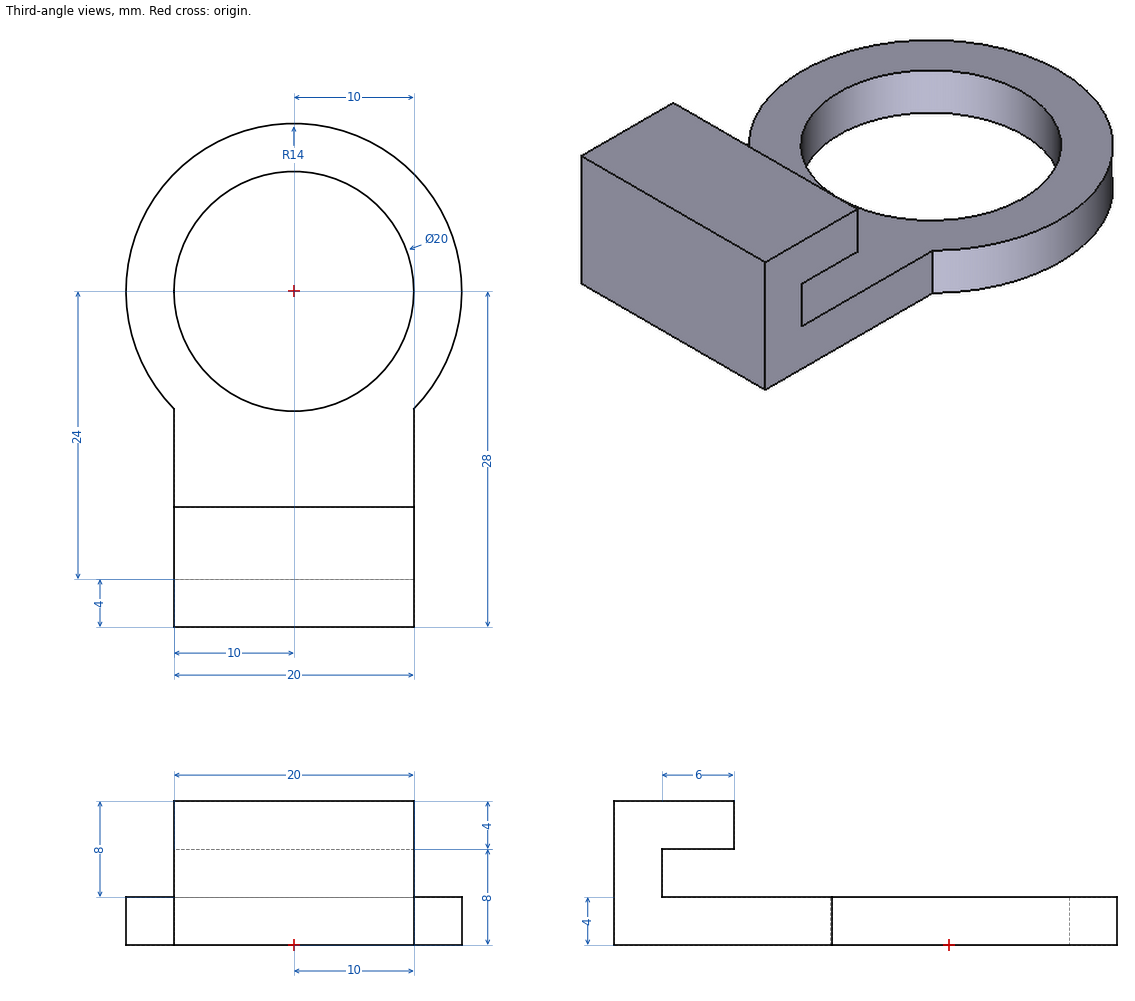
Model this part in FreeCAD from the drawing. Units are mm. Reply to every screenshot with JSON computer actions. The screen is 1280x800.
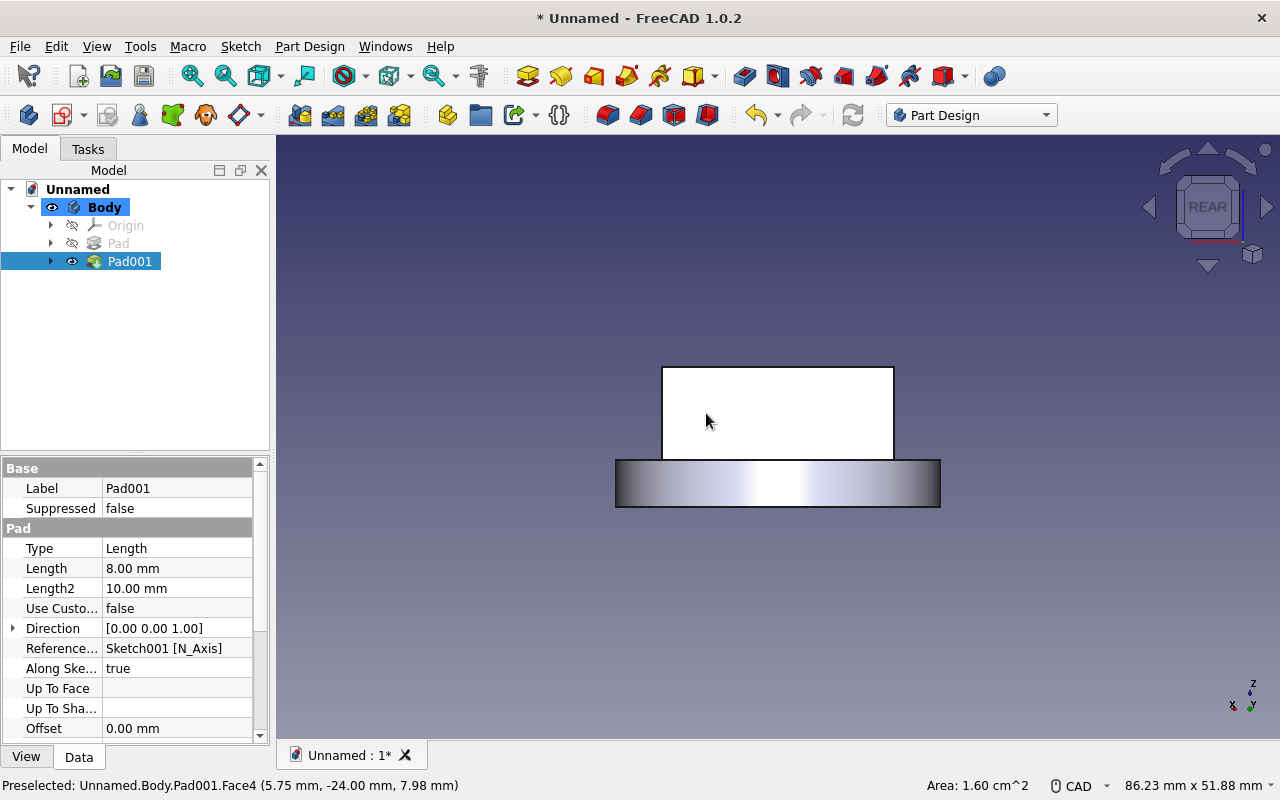
{"action": "left_click", "coordinate": [62, 116]}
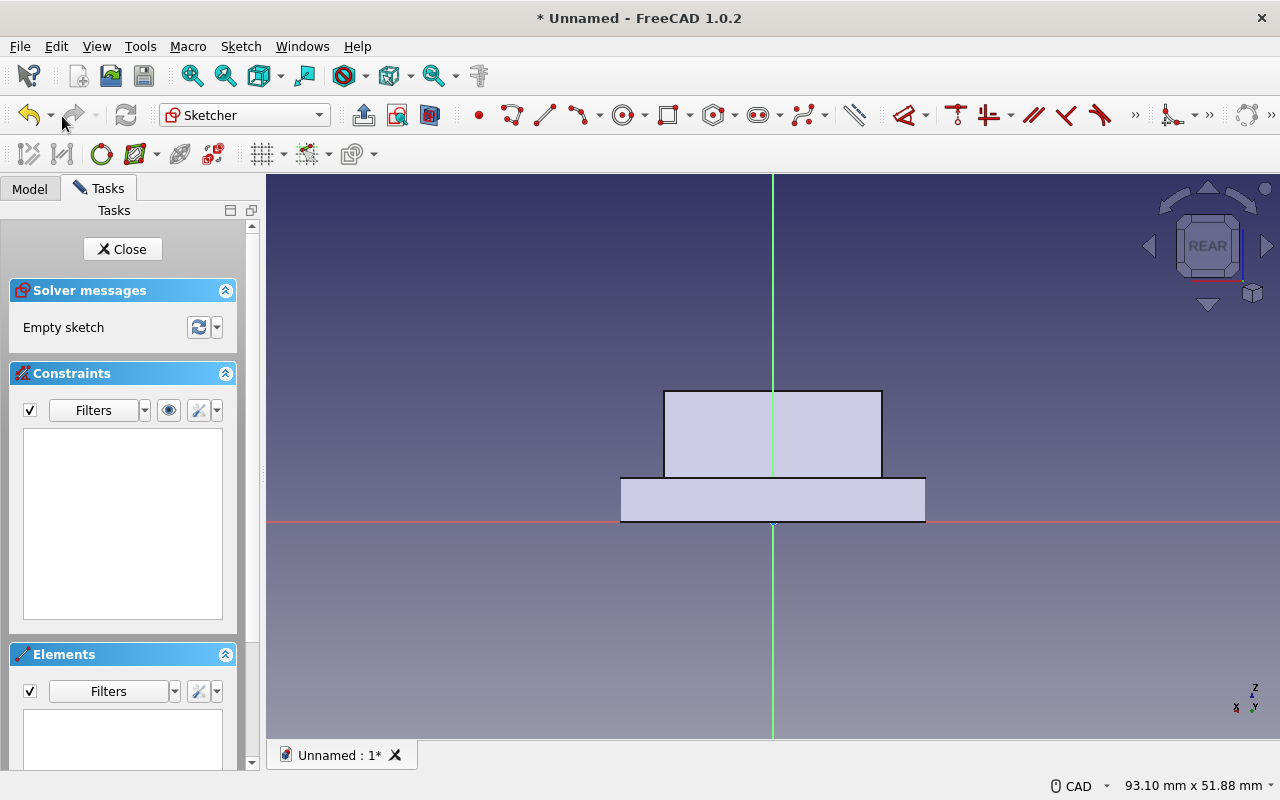
{"action": "left_click", "coordinate": [430, 116]}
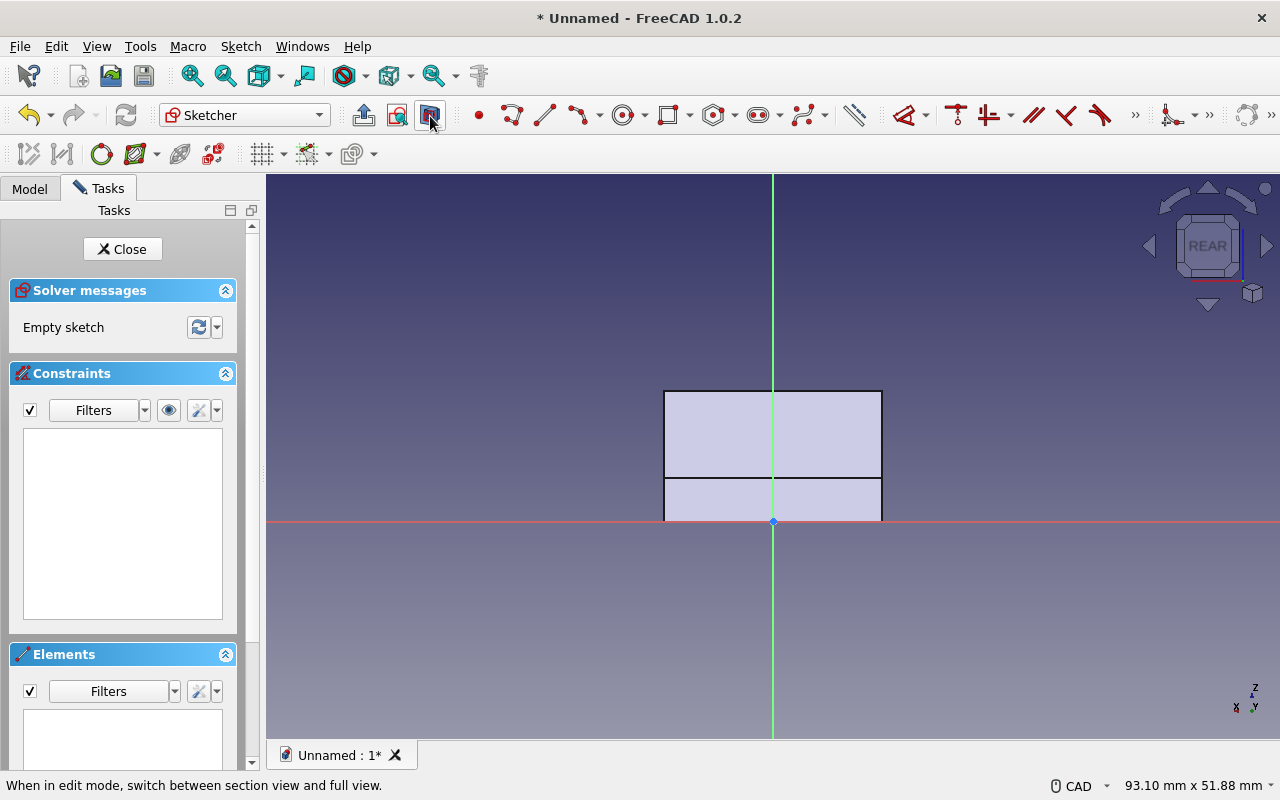
{"action": "scroll", "coordinate": [813, 456], "scroll_direction": "up", "scroll_amount": 5}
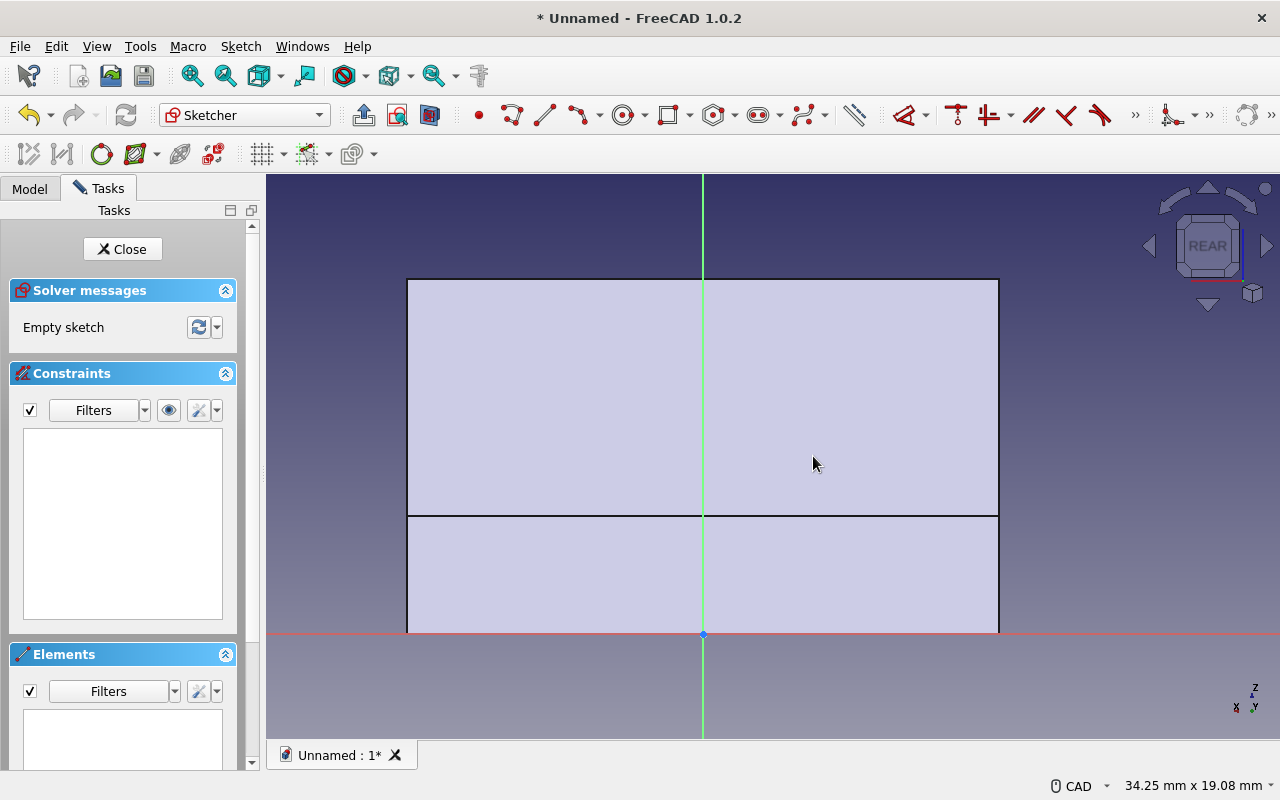
{"action": "left_click", "coordinate": [668, 116]}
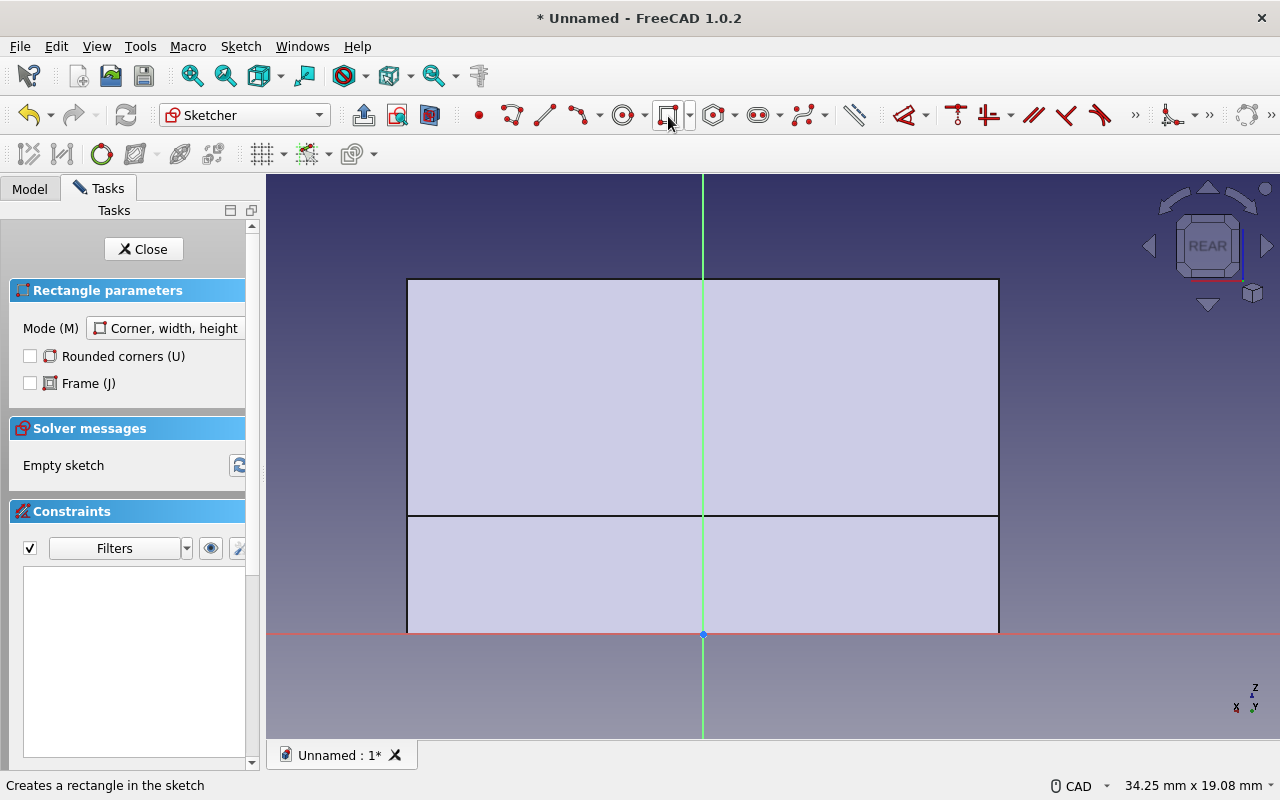
{"action": "left_click", "coordinate": [407, 279]}
{"action": "left_click", "coordinate": [999, 397]}
{"action": "key", "text": "Escape"}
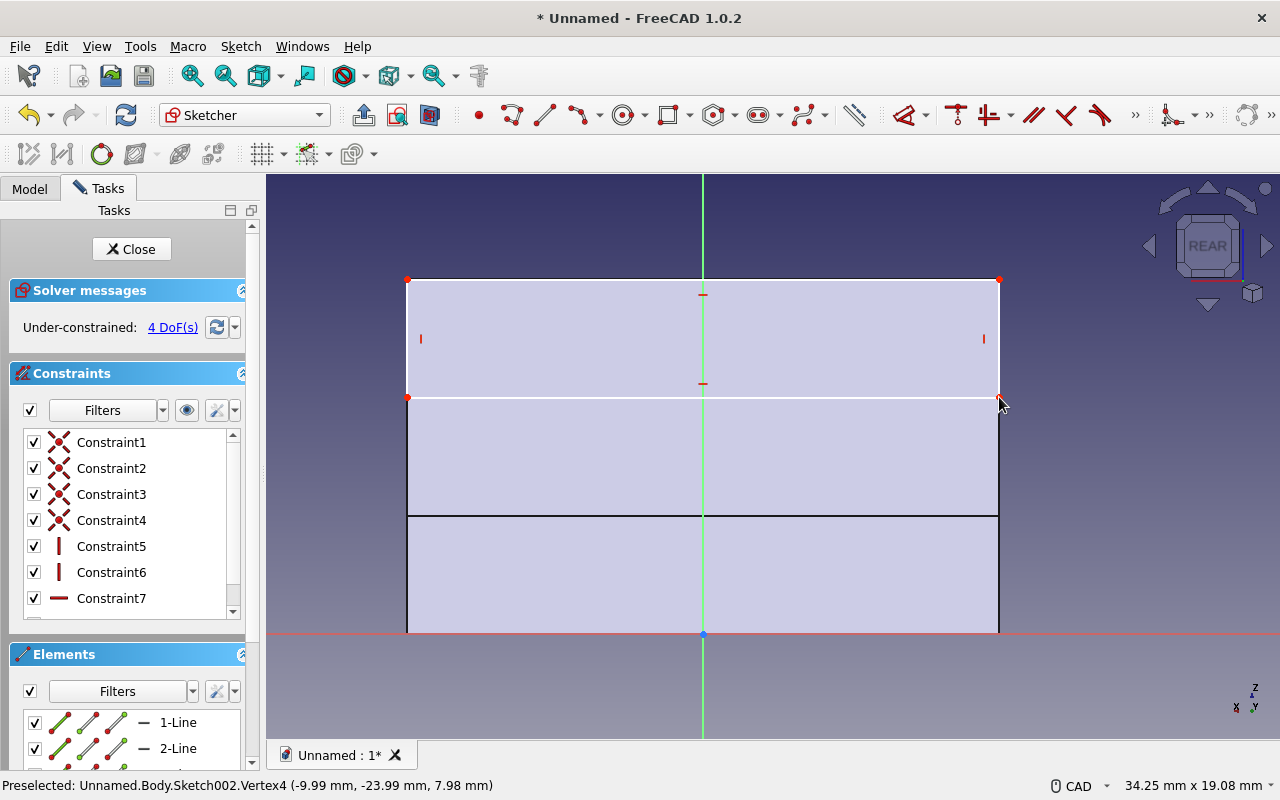
{"action": "key", "text": "d"}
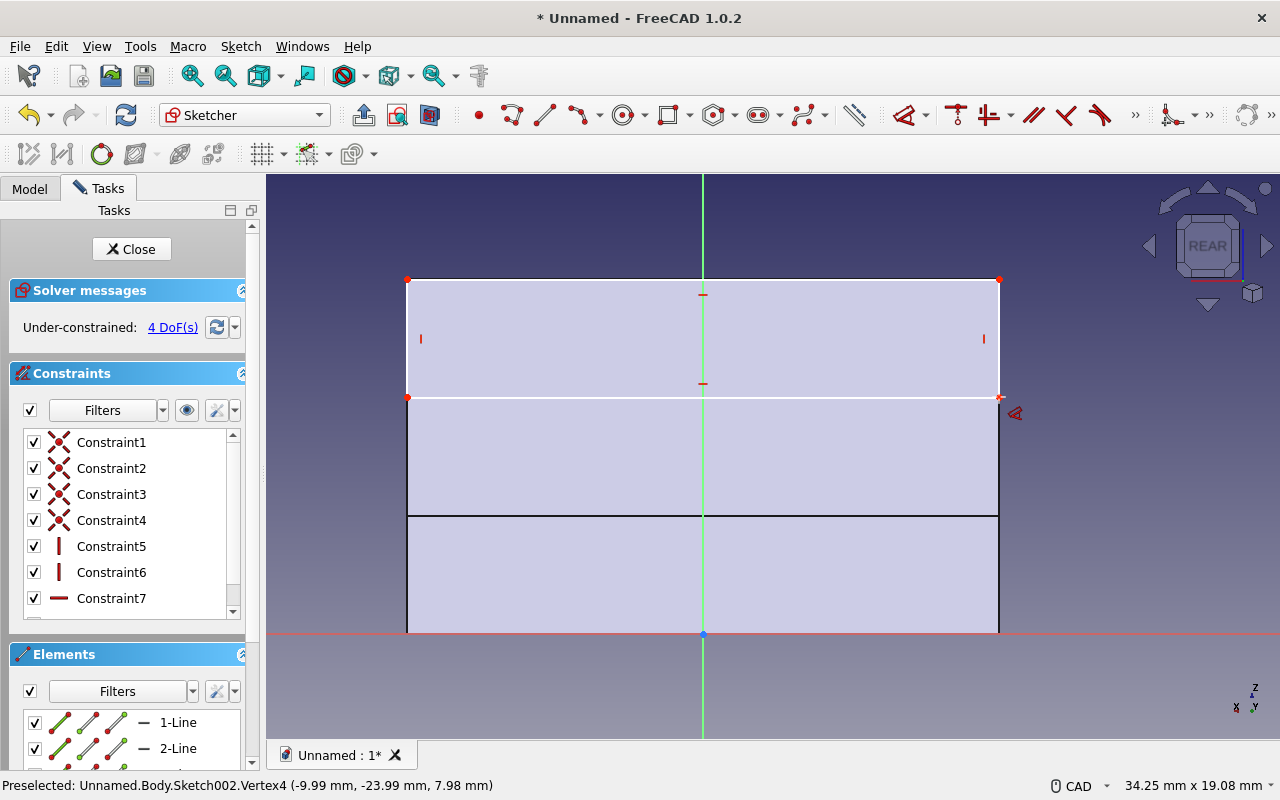
{"action": "left_click", "coordinate": [407, 315]}
{"action": "left_click", "coordinate": [373, 339]}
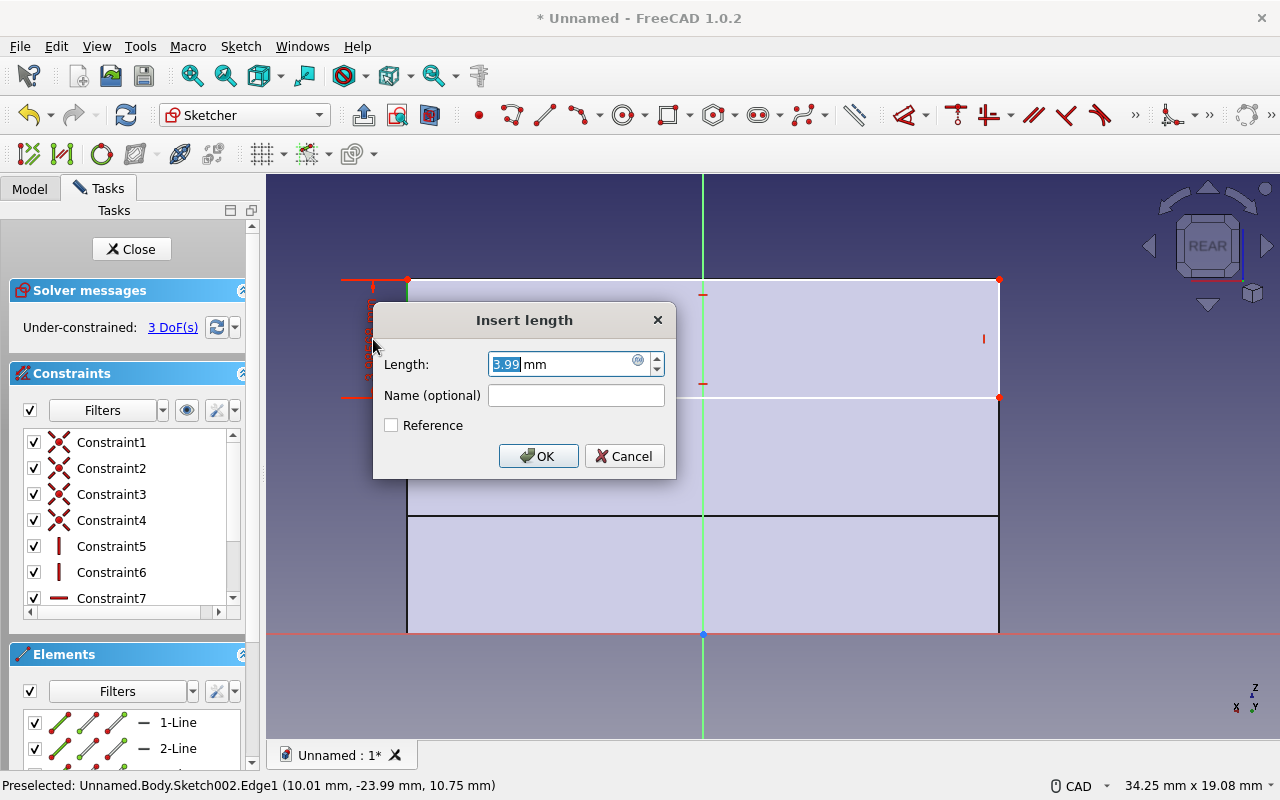
{"action": "type", "text": "4"}
{"action": "key", "text": "Return"}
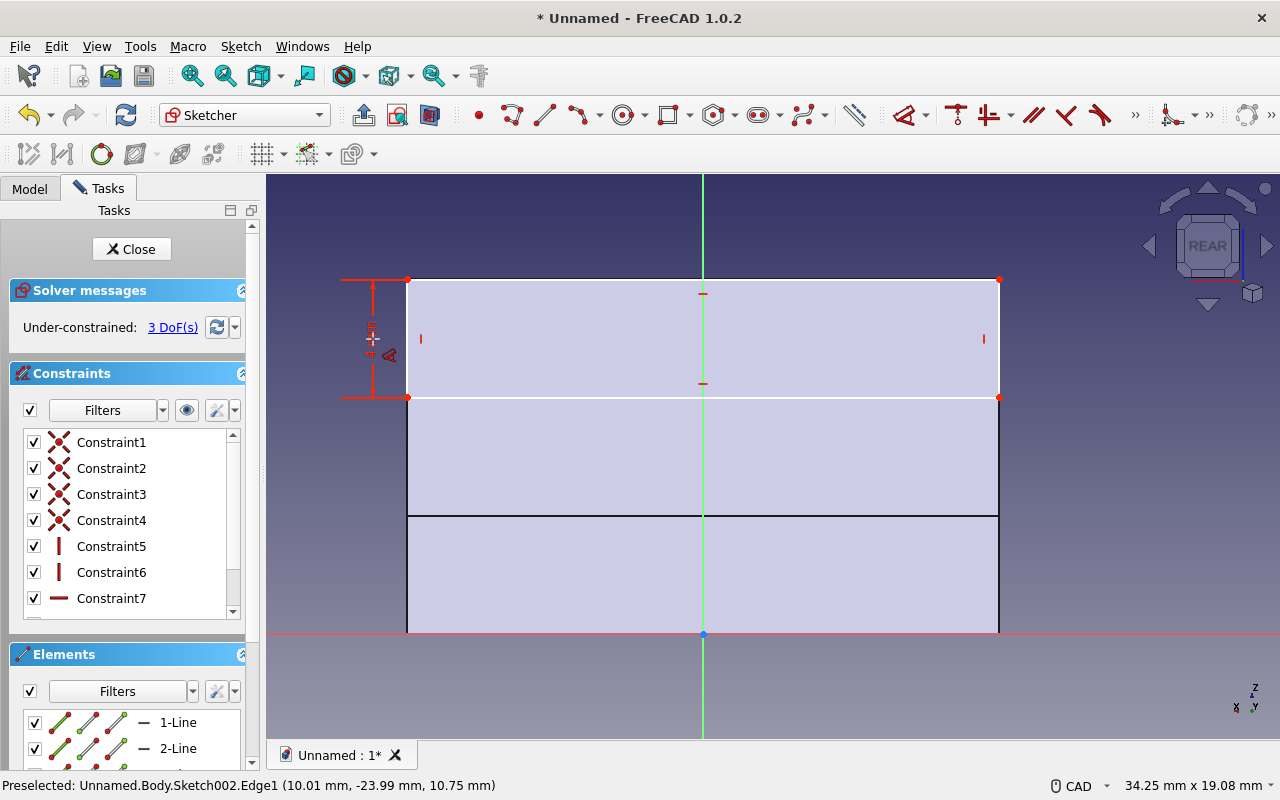
{"action": "left_click", "coordinate": [585, 398]}
{"action": "left_click", "coordinate": [567, 364]}